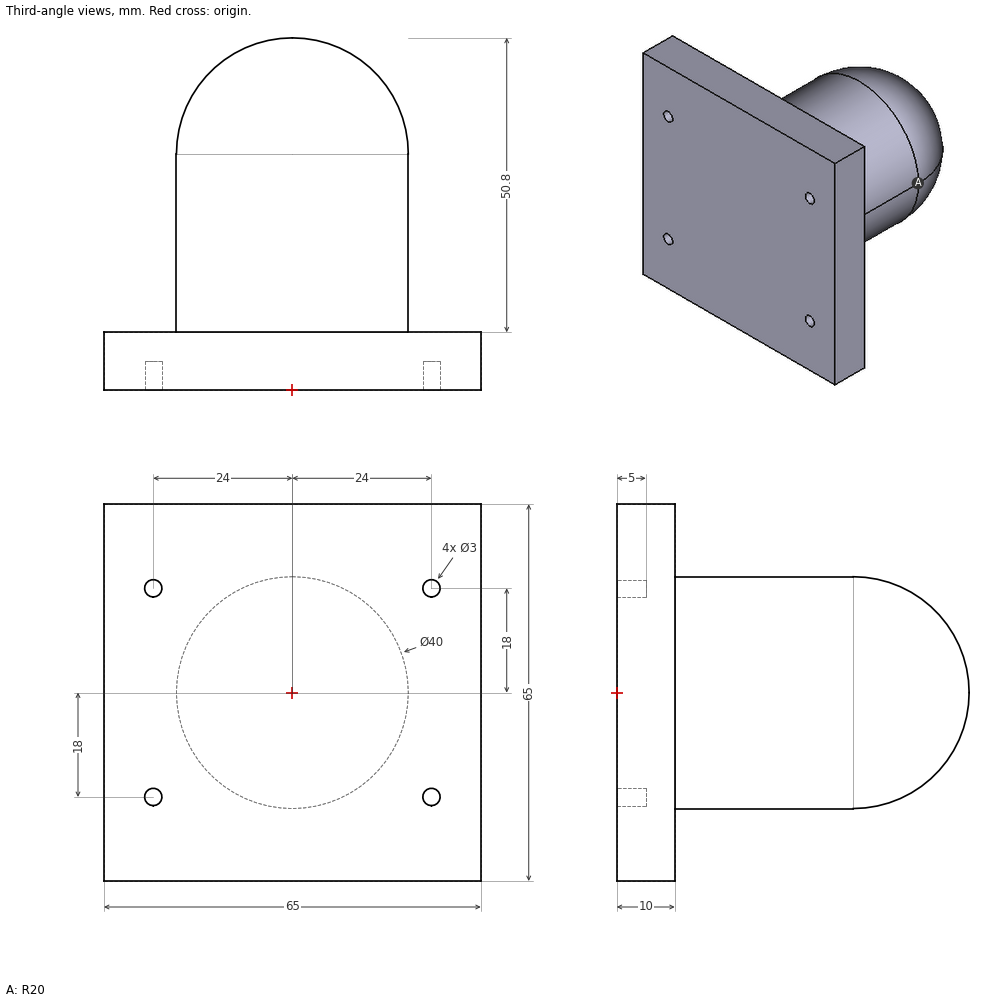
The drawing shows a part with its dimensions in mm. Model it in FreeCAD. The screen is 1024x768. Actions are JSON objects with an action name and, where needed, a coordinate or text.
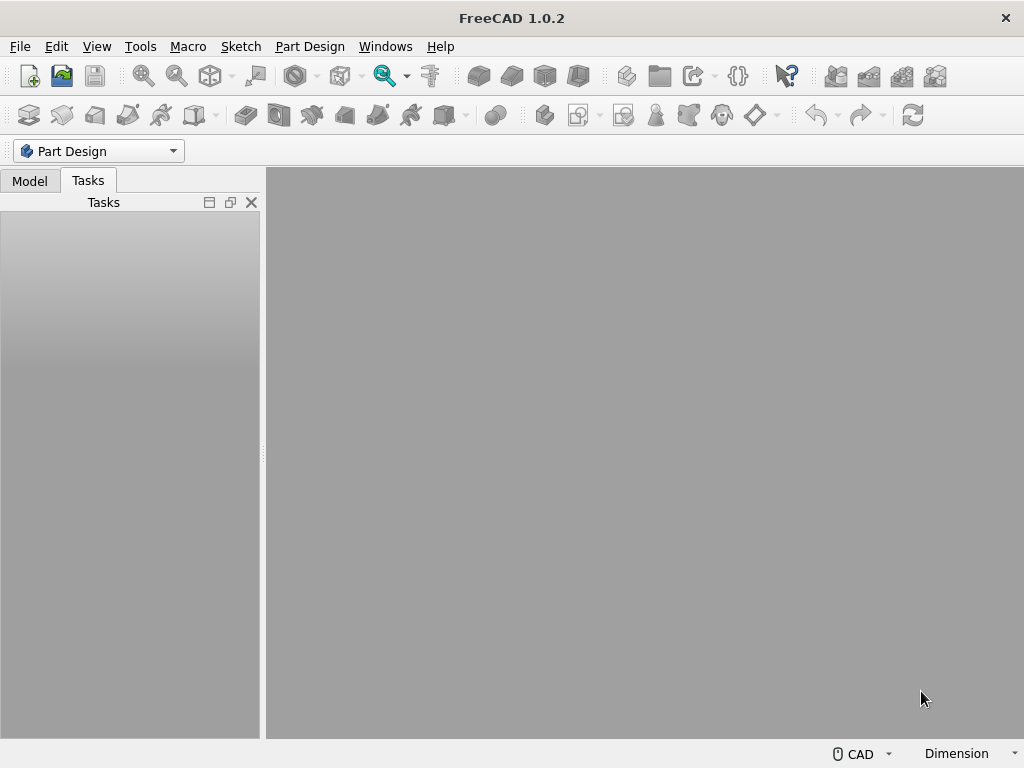
{"action": "left_click", "coordinate": [29, 76]}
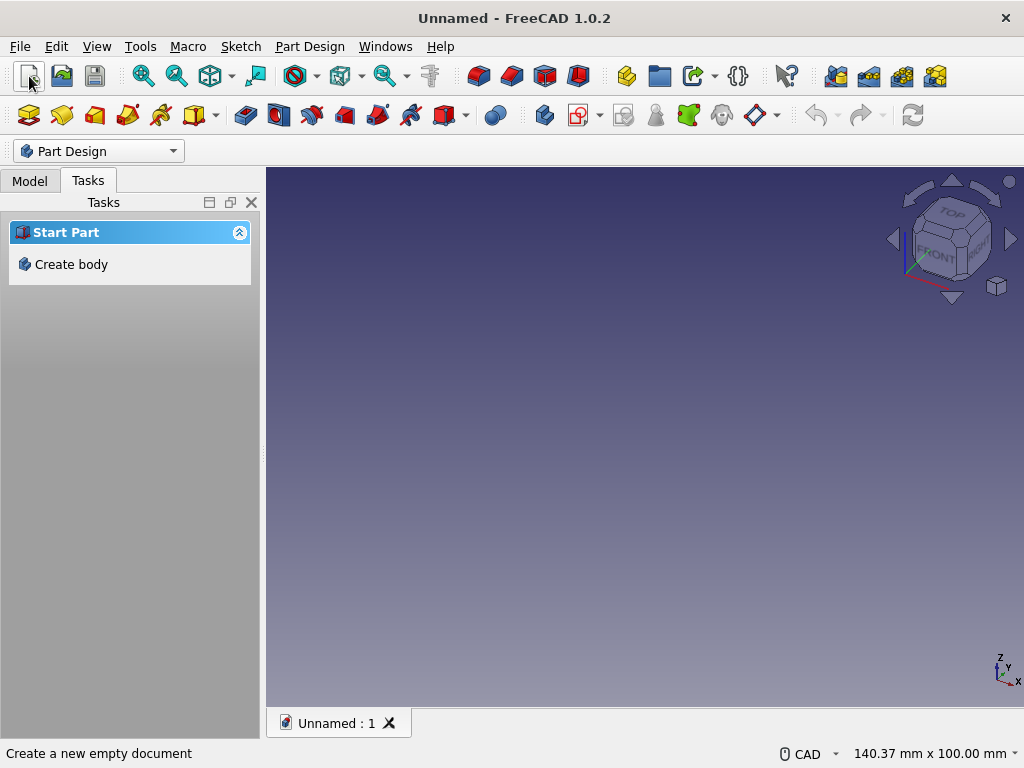
{"action": "left_click", "coordinate": [578, 116]}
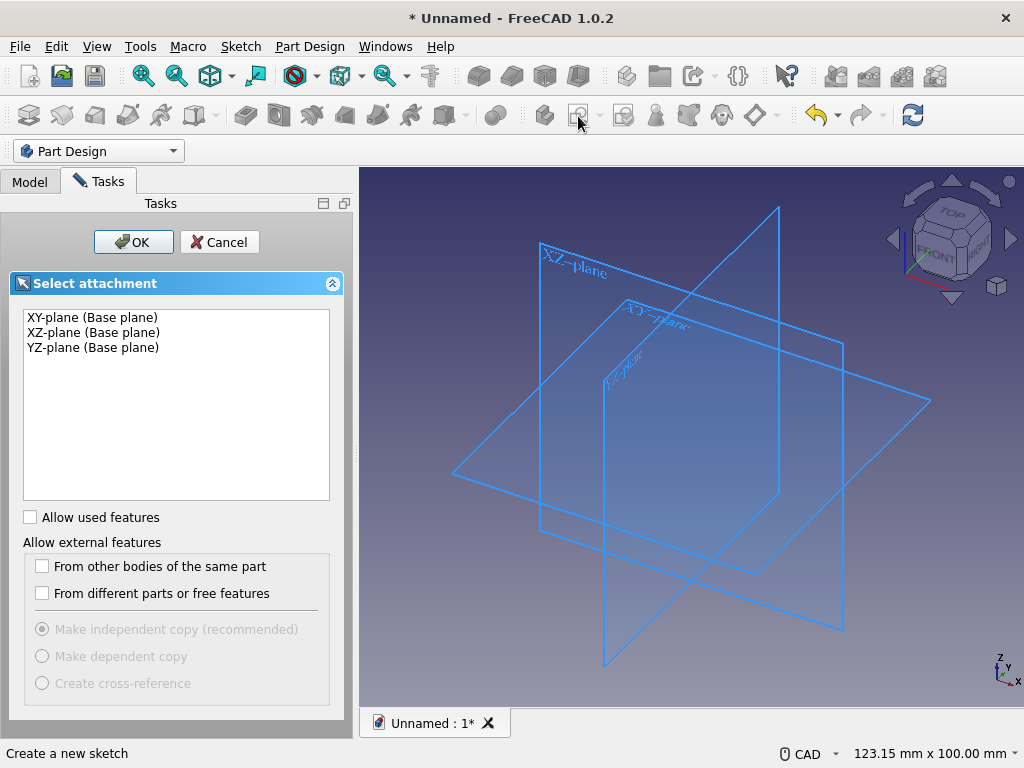
{"action": "left_click", "coordinate": [84, 332]}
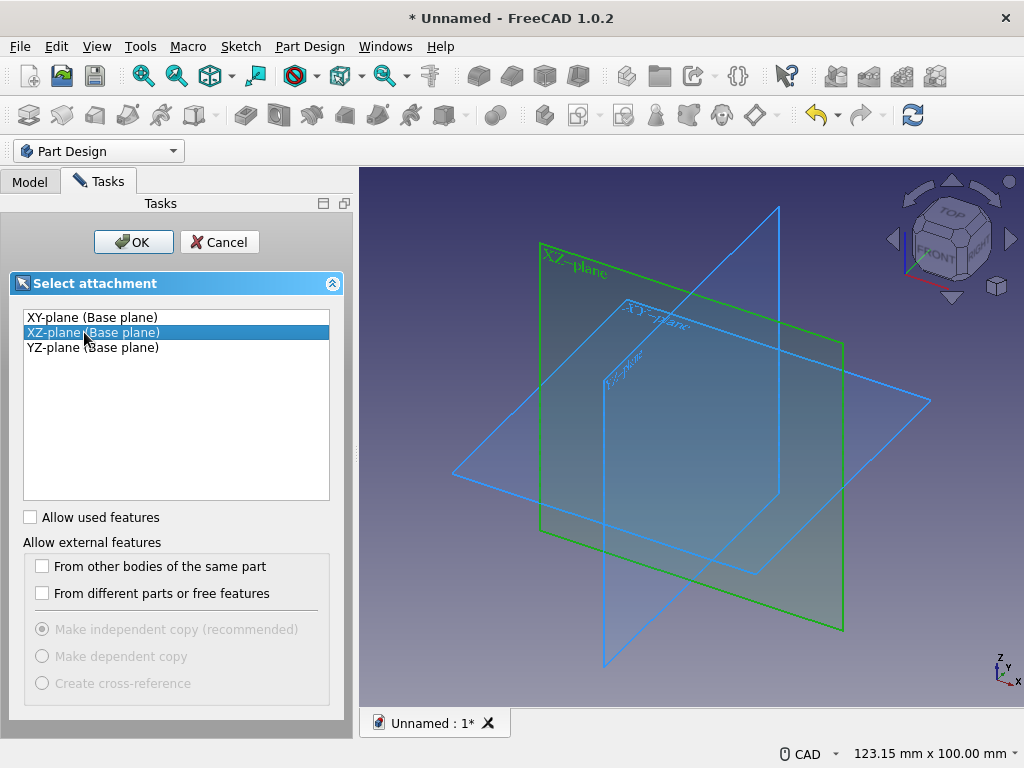
{"action": "left_click", "coordinate": [134, 242]}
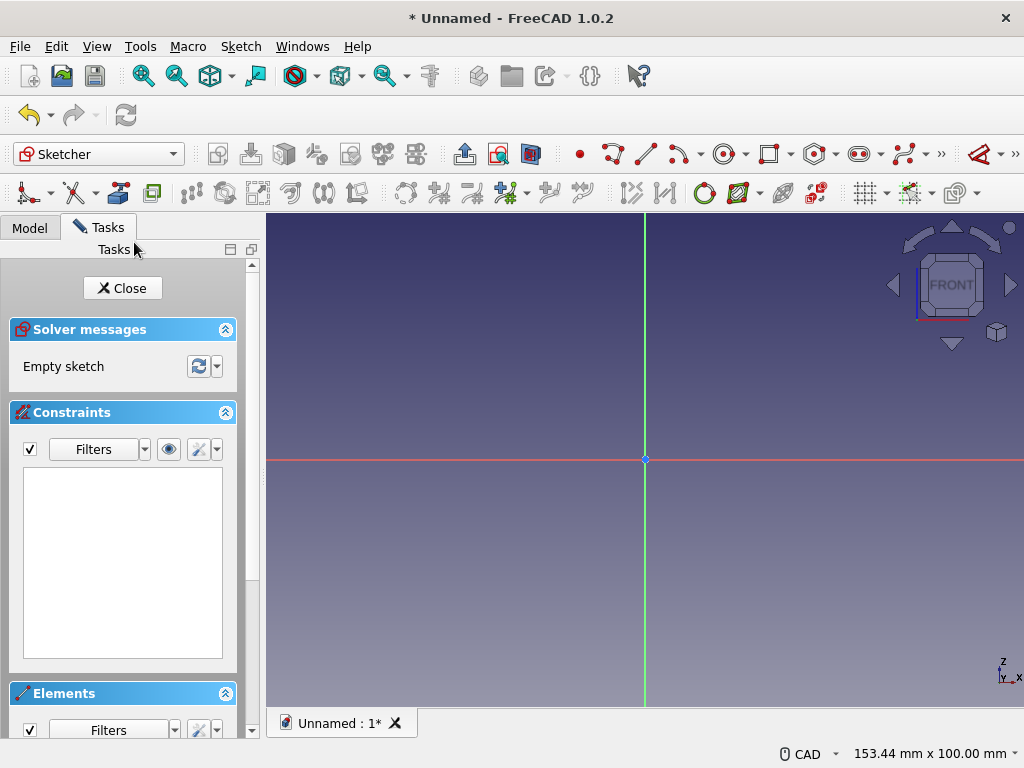
{"action": "key", "text": "g v"}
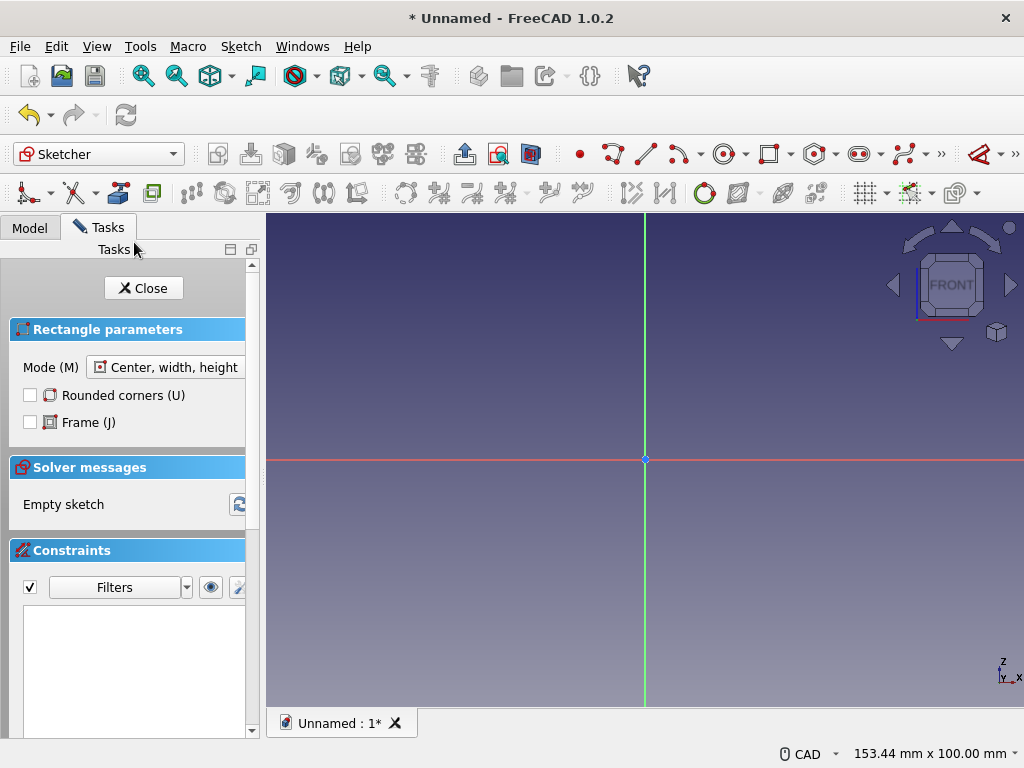
{"action": "left_click", "coordinate": [645, 460]}
{"action": "mouse_move", "coordinate": [806, 299]}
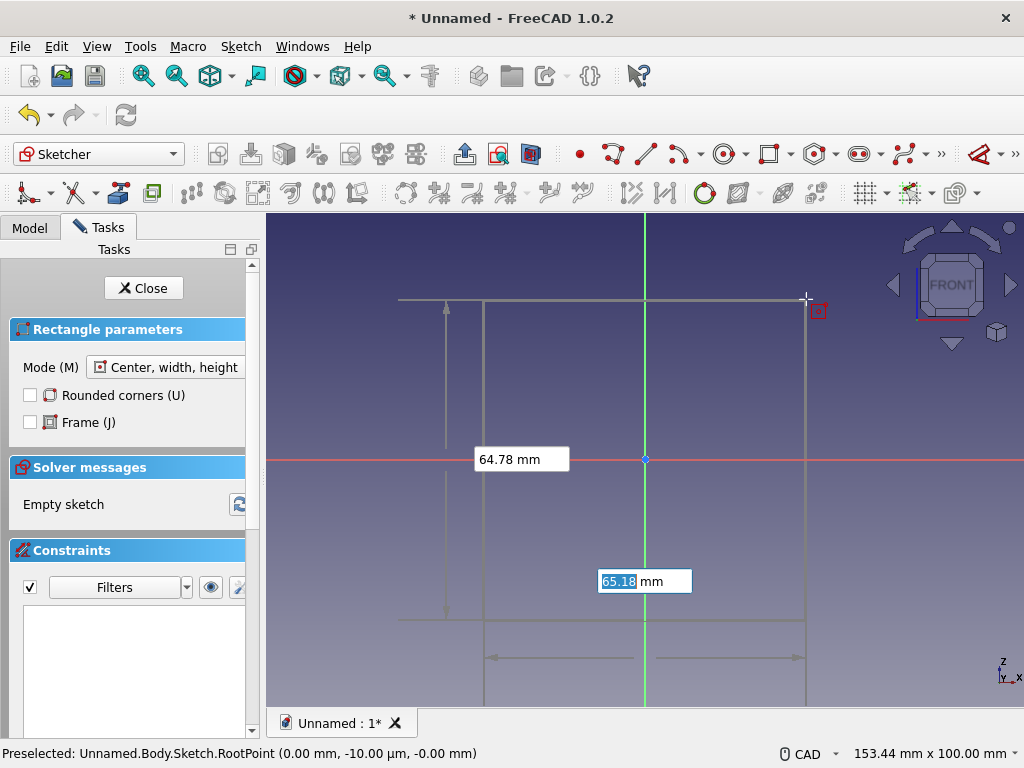
{"action": "type", "text": "65"}
{"action": "key", "text": "Tab"}
{"action": "type", "text": "65"}
{"action": "key", "text": "Return"}
{"action": "key", "text": "Escape"}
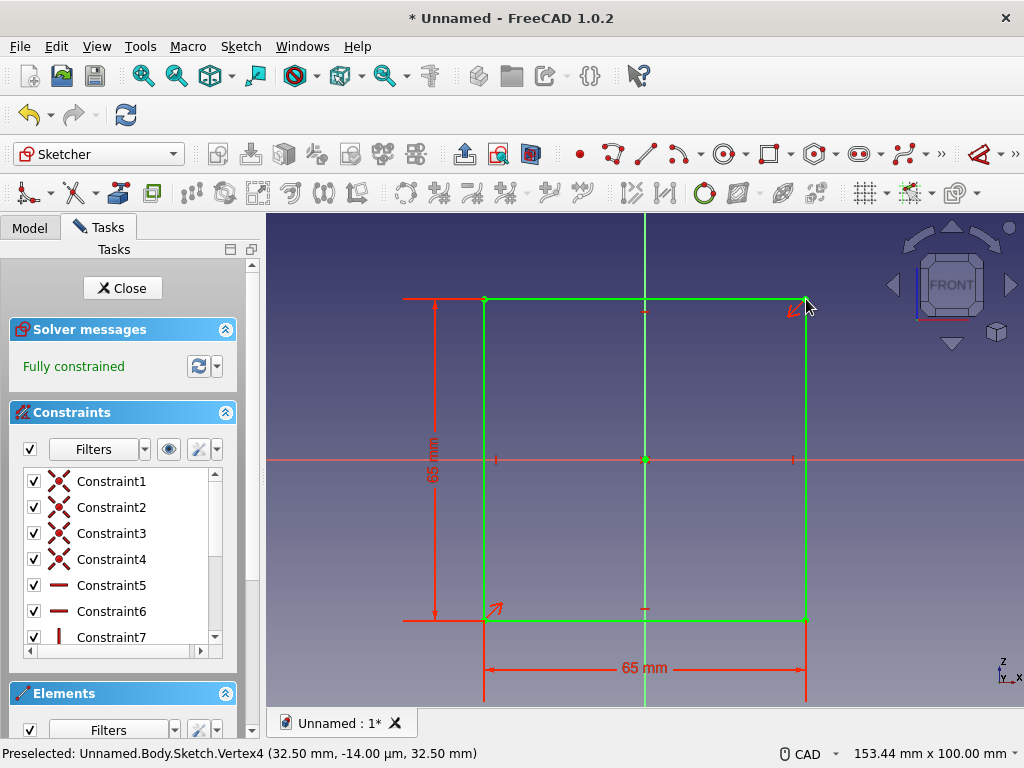
{"action": "left_click", "coordinate": [123, 288]}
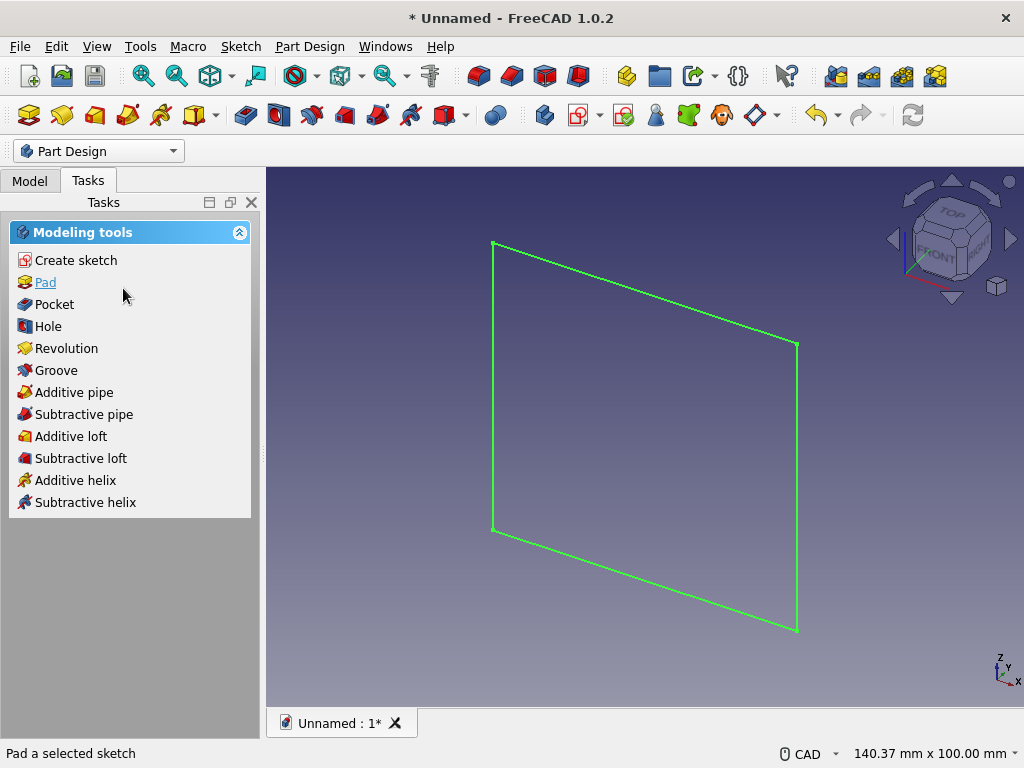
{"action": "left_click", "coordinate": [29, 116]}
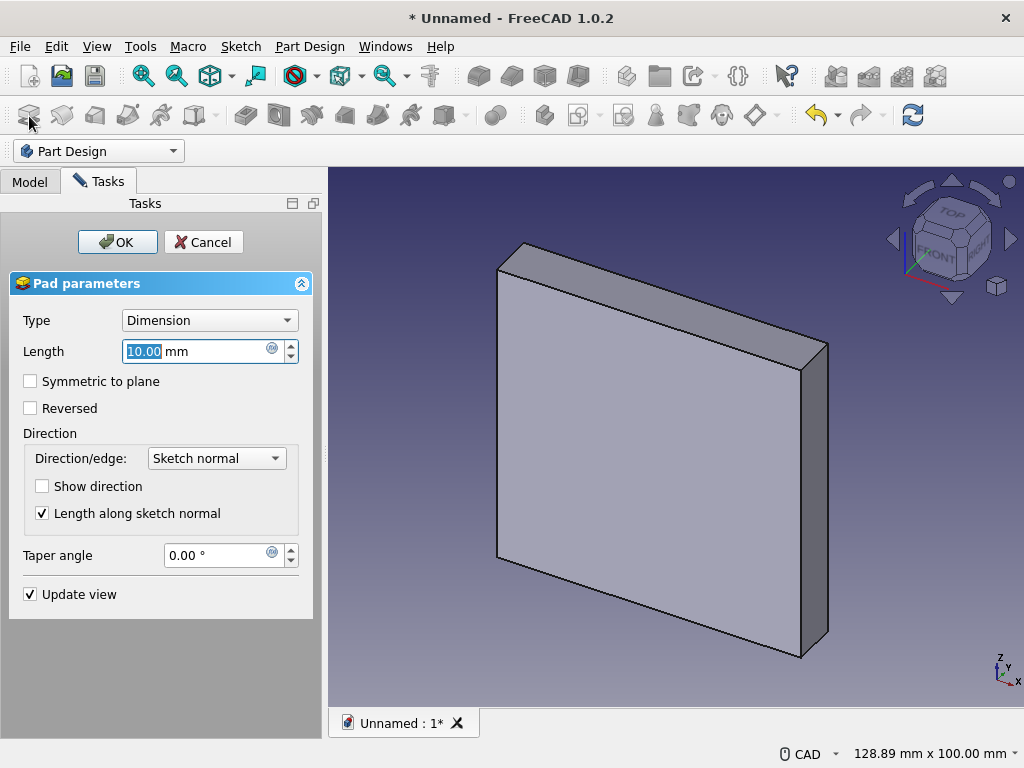
{"action": "type", "text": "10"}
{"action": "key", "text": "Tab"}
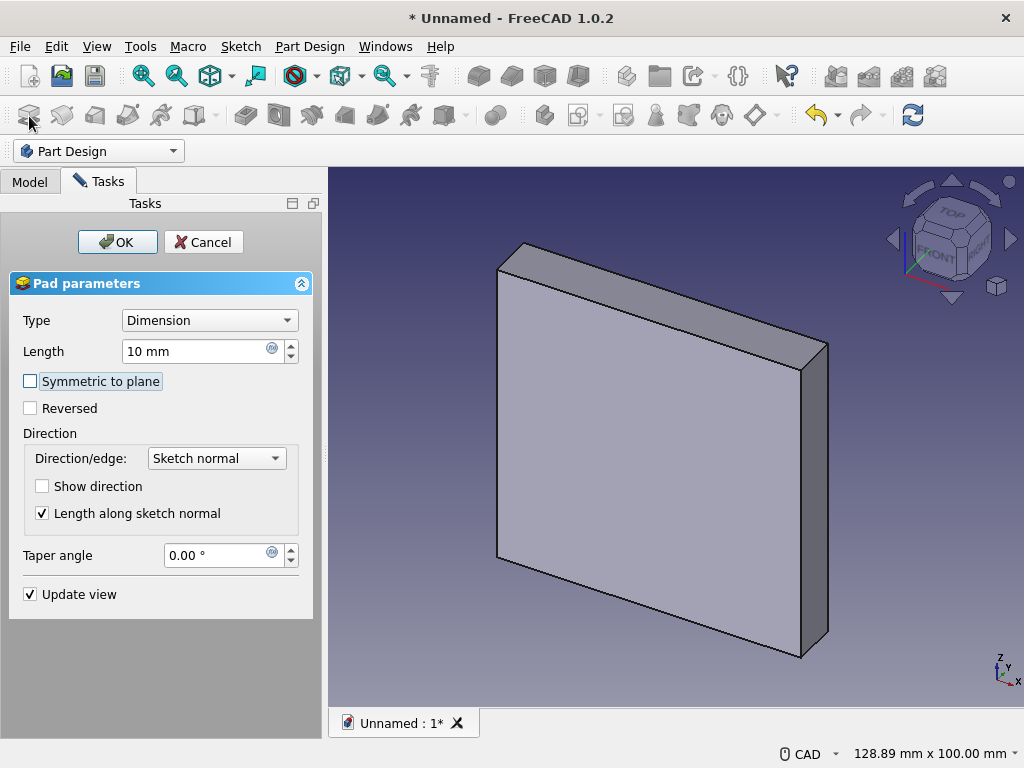
{"action": "left_click", "coordinate": [31, 408]}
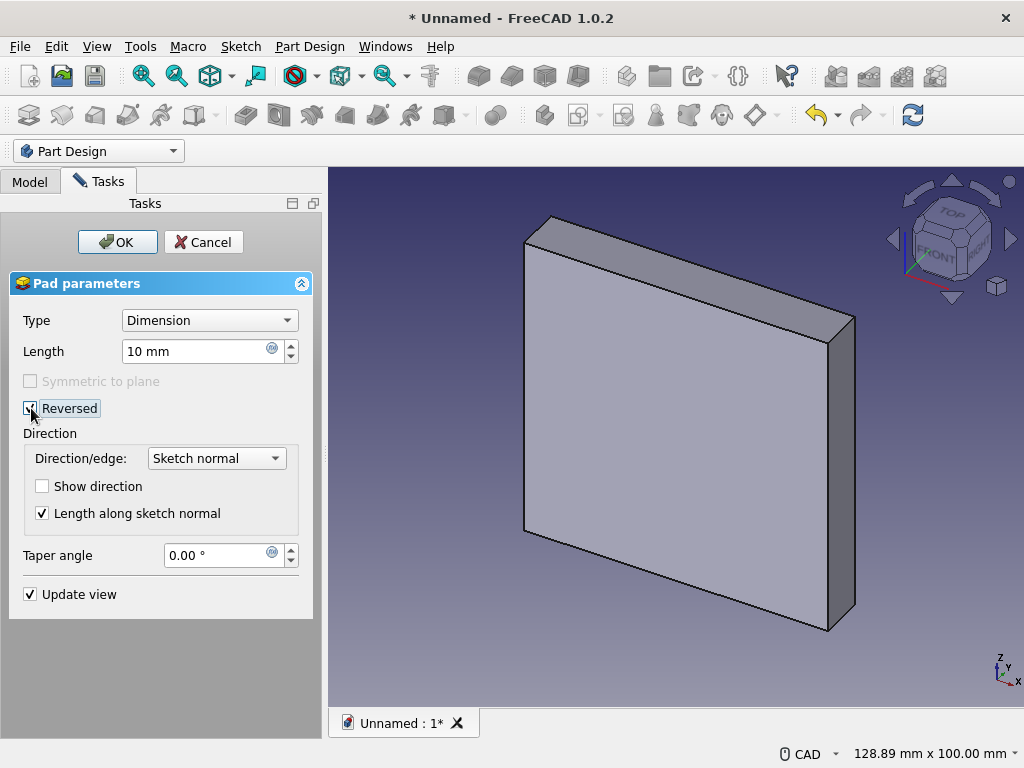
{"action": "left_click", "coordinate": [118, 242]}